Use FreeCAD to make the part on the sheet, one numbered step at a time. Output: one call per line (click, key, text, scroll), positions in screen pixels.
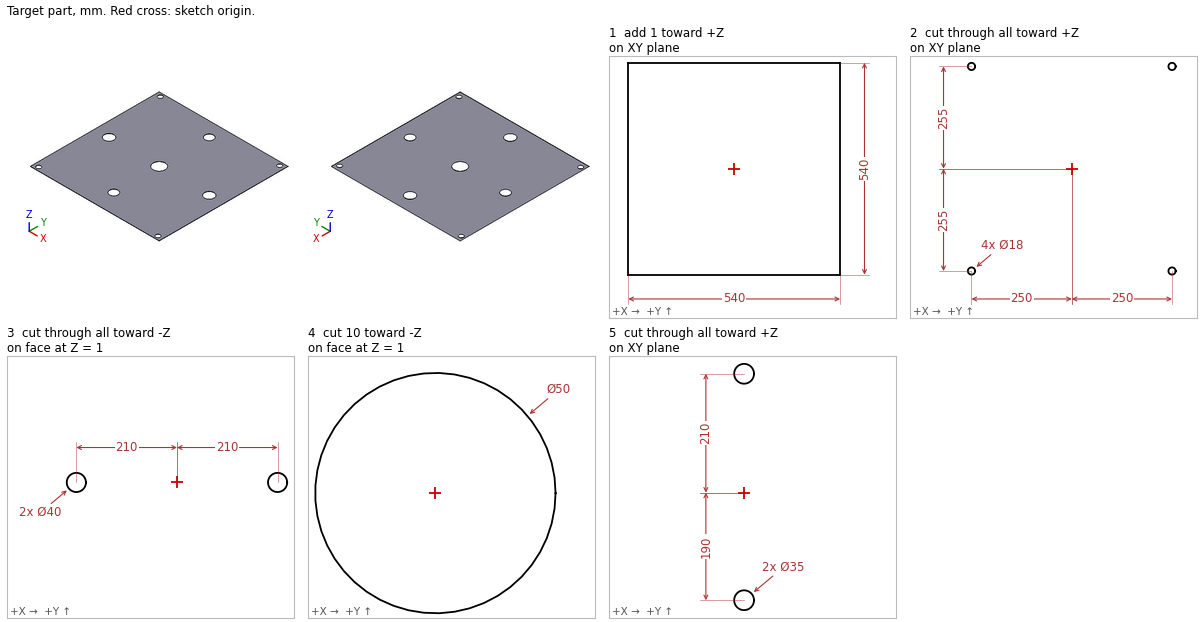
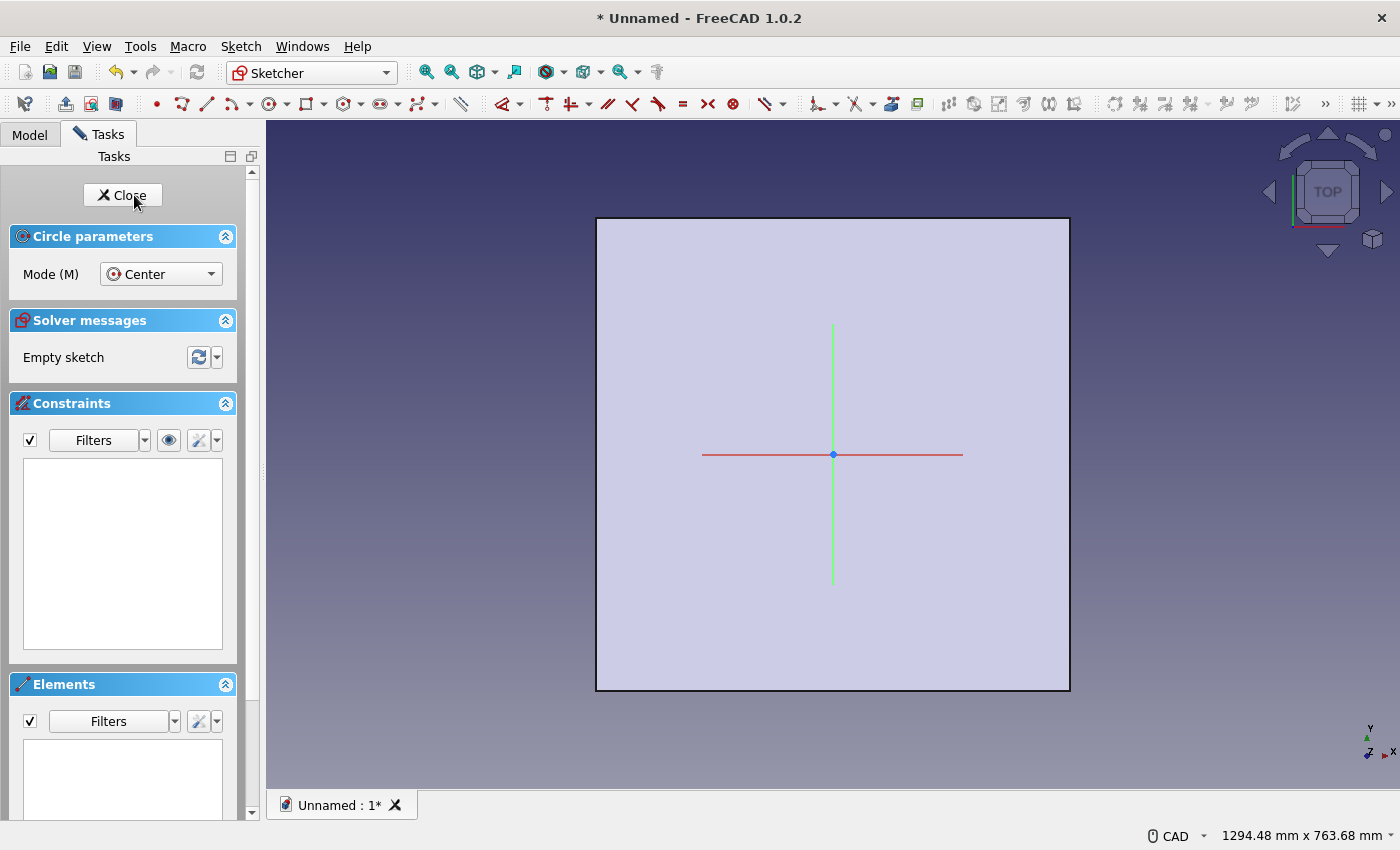
scroll(614, 678, up, 6)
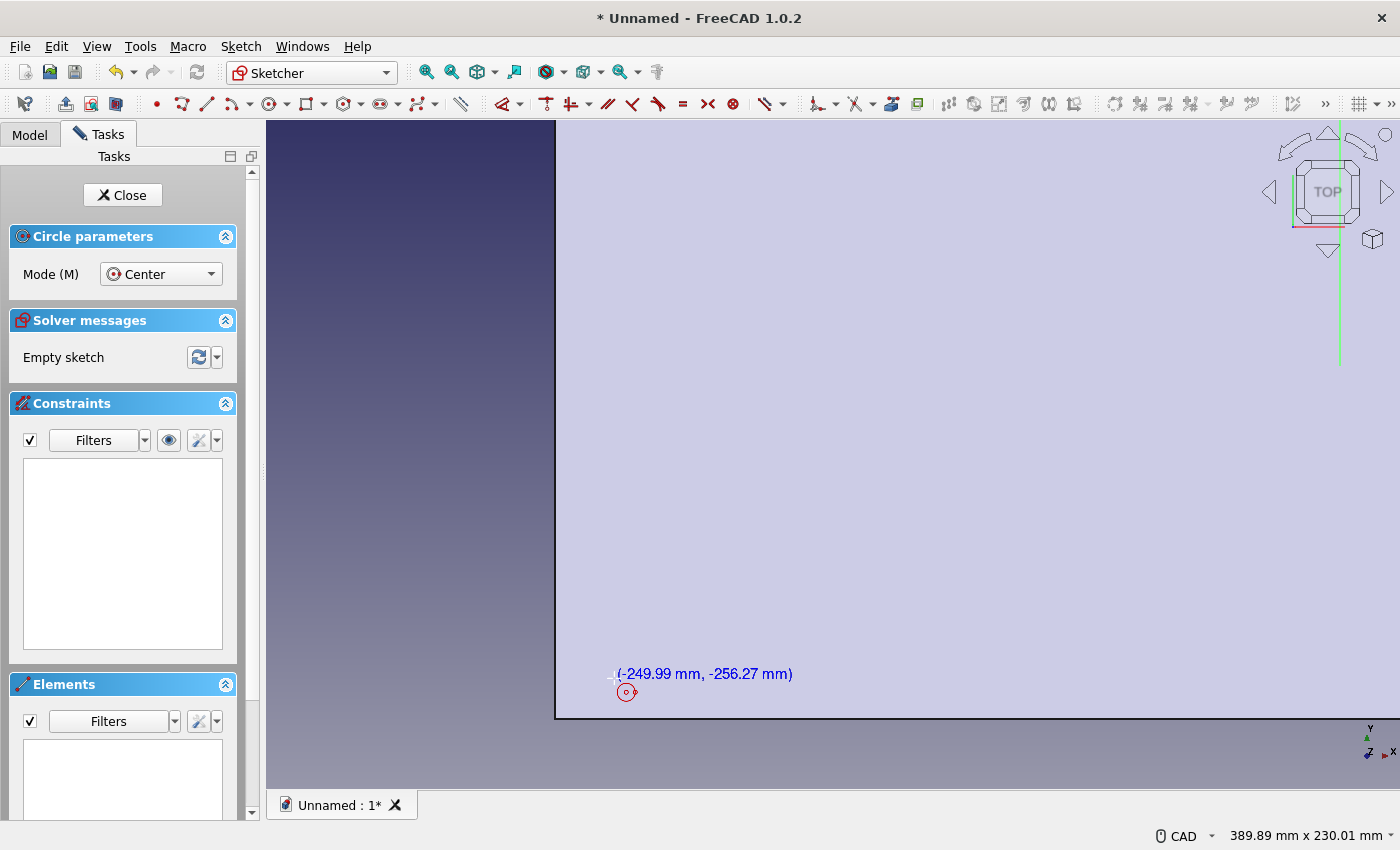
click(613, 676)
move(632, 657)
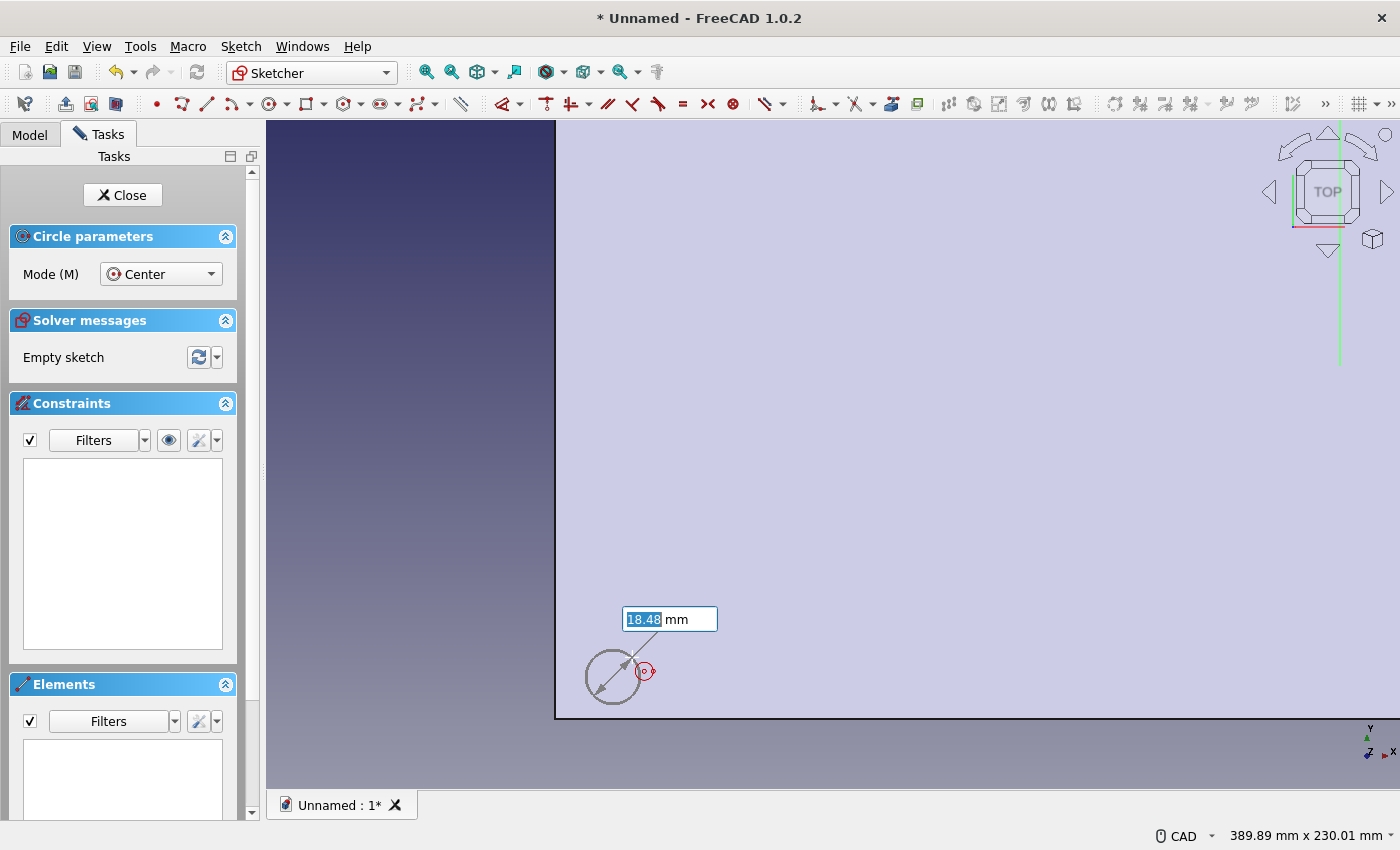
text(18)
key(Return)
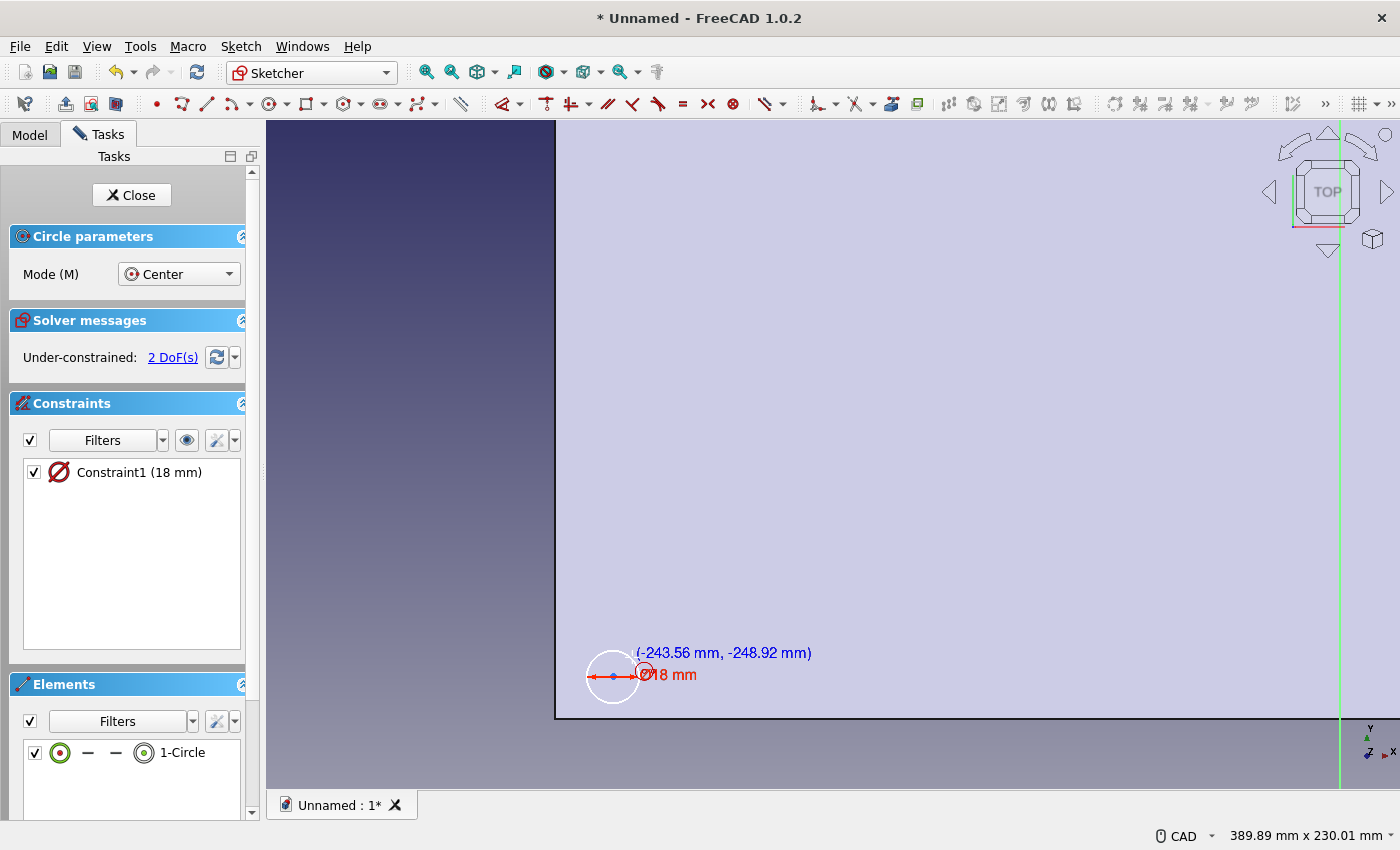
scroll(516, 679, down, 6)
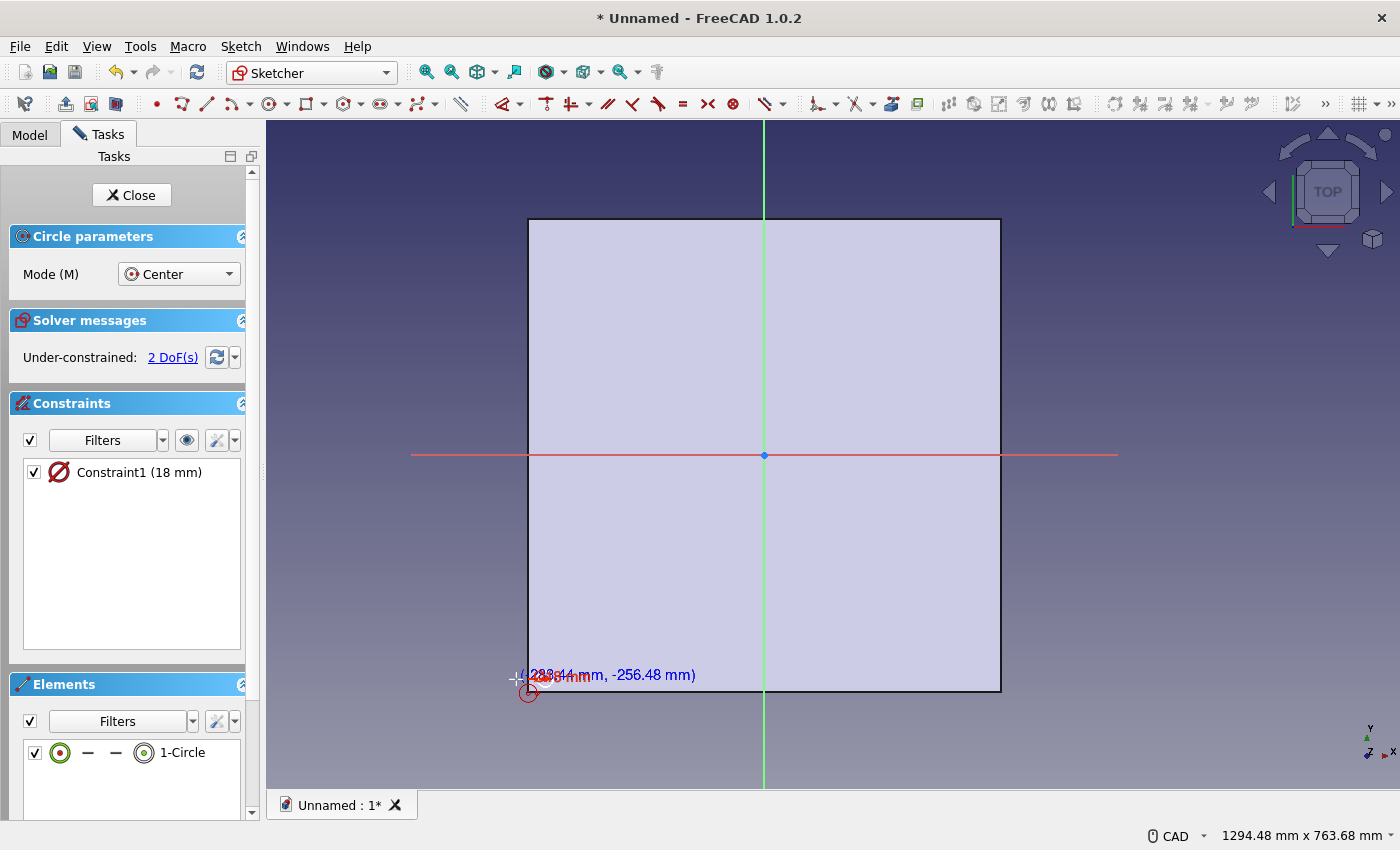
scroll(983, 679, up, 6)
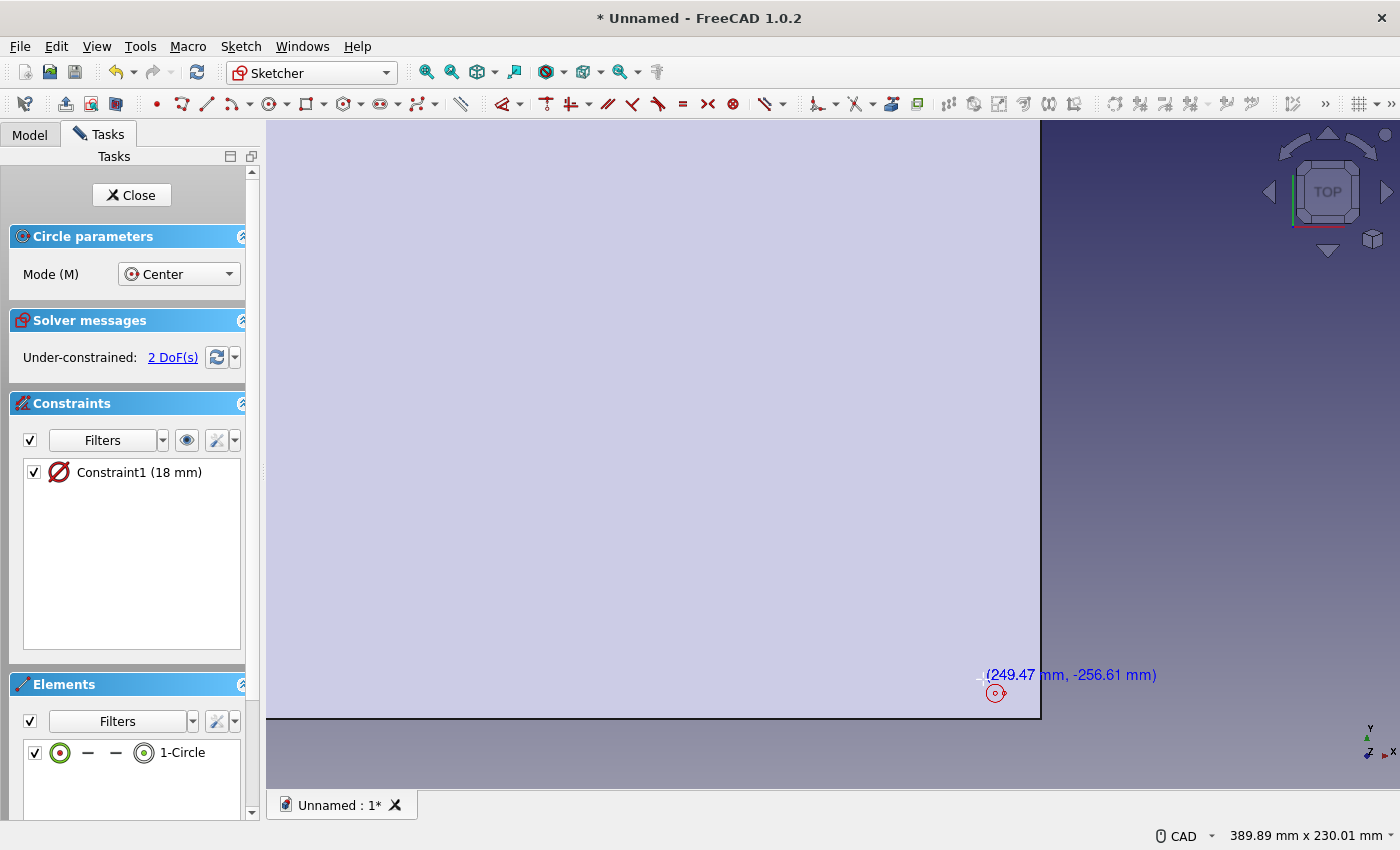
click(983, 676)
move(1002, 657)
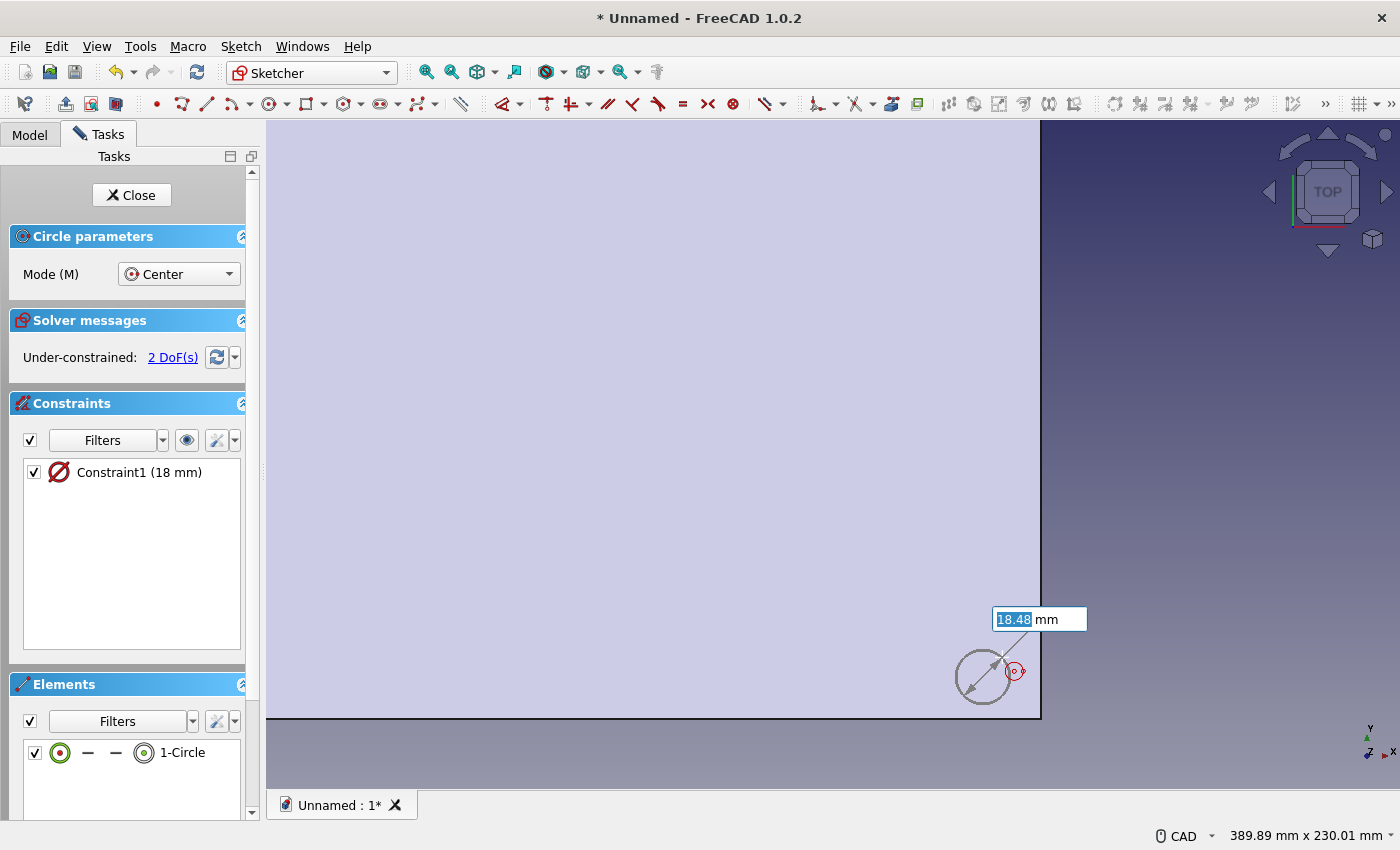
text(18)
key(Return)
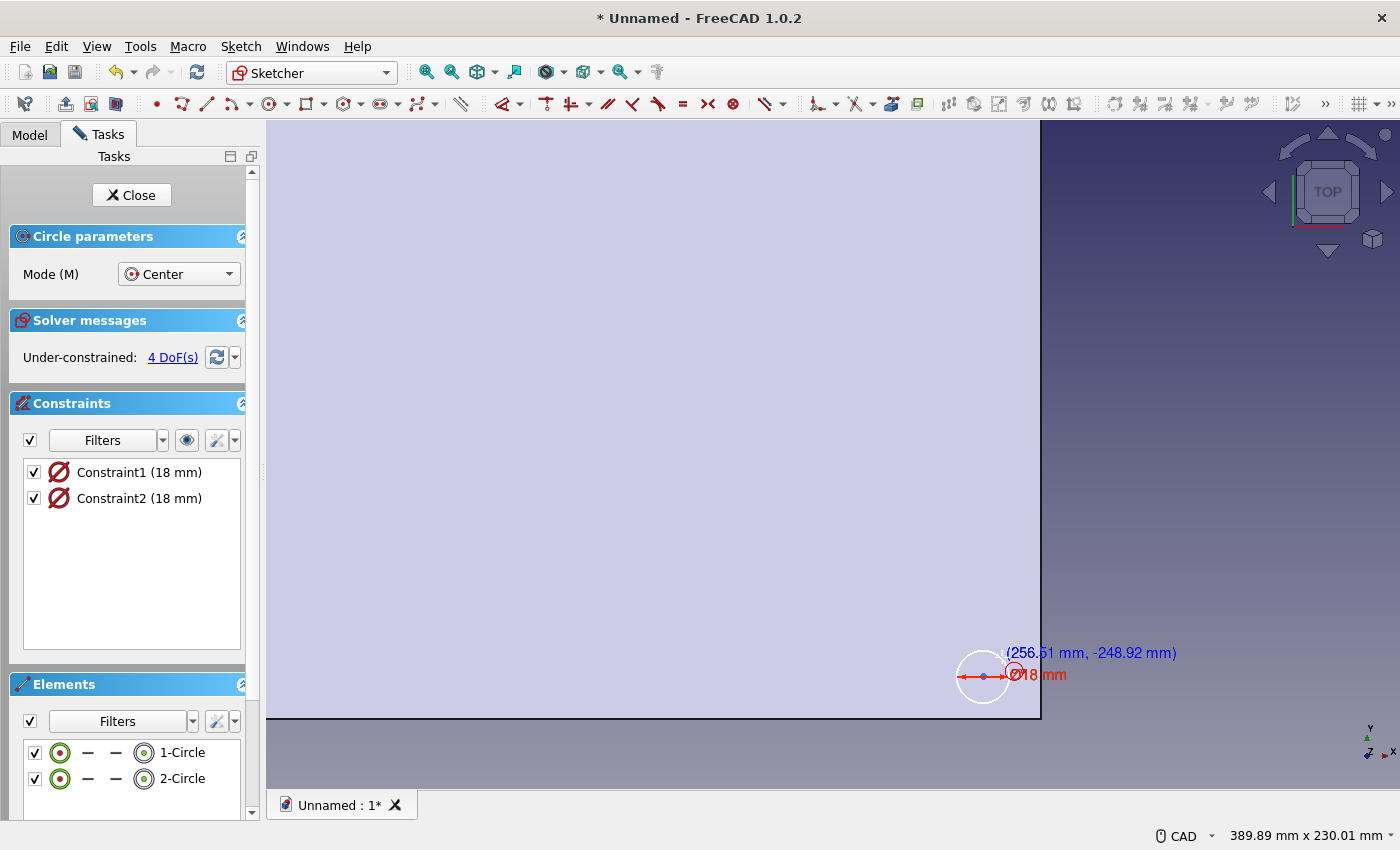
scroll(984, 679, down, 6)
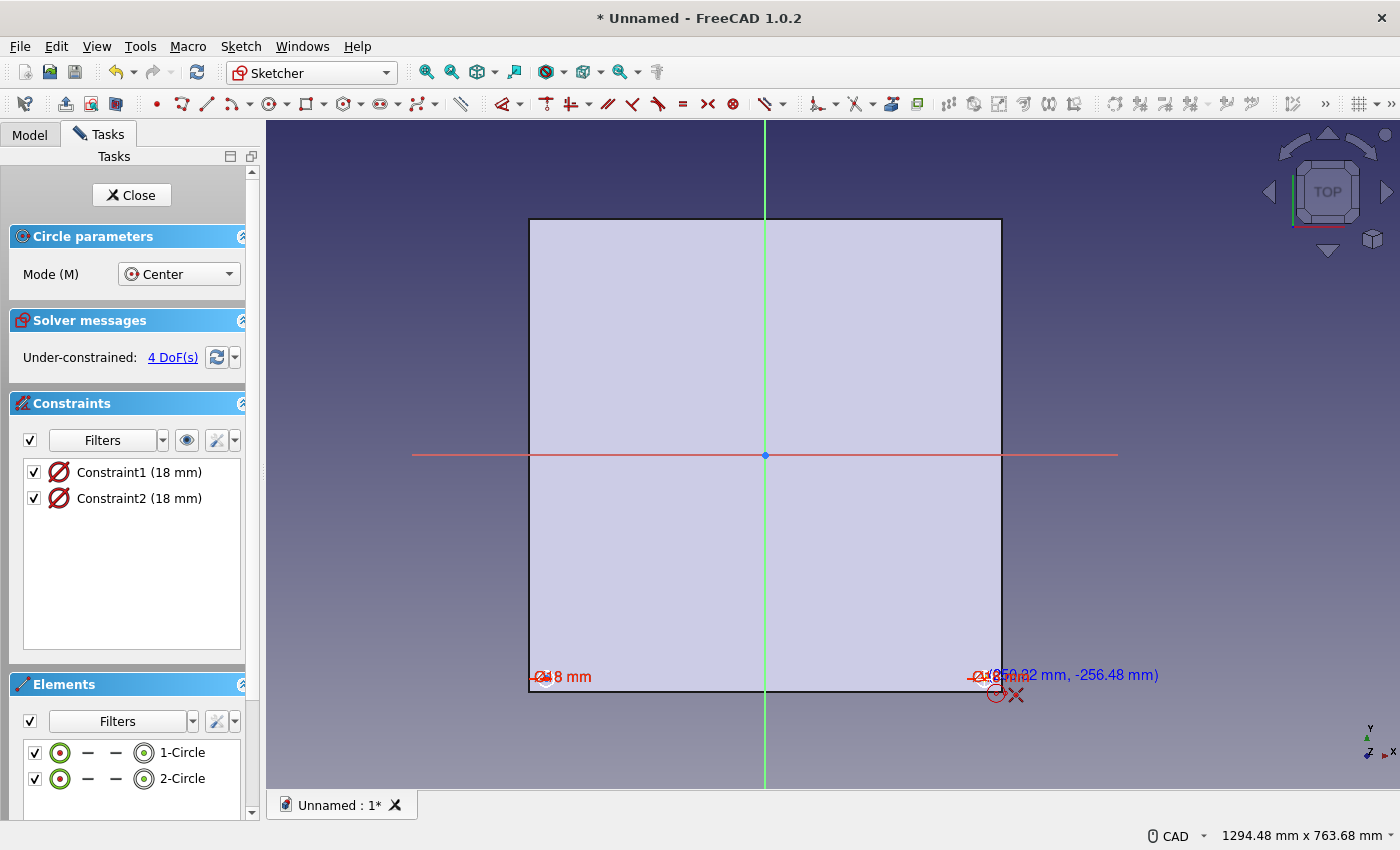
scroll(546, 232, up, 6)